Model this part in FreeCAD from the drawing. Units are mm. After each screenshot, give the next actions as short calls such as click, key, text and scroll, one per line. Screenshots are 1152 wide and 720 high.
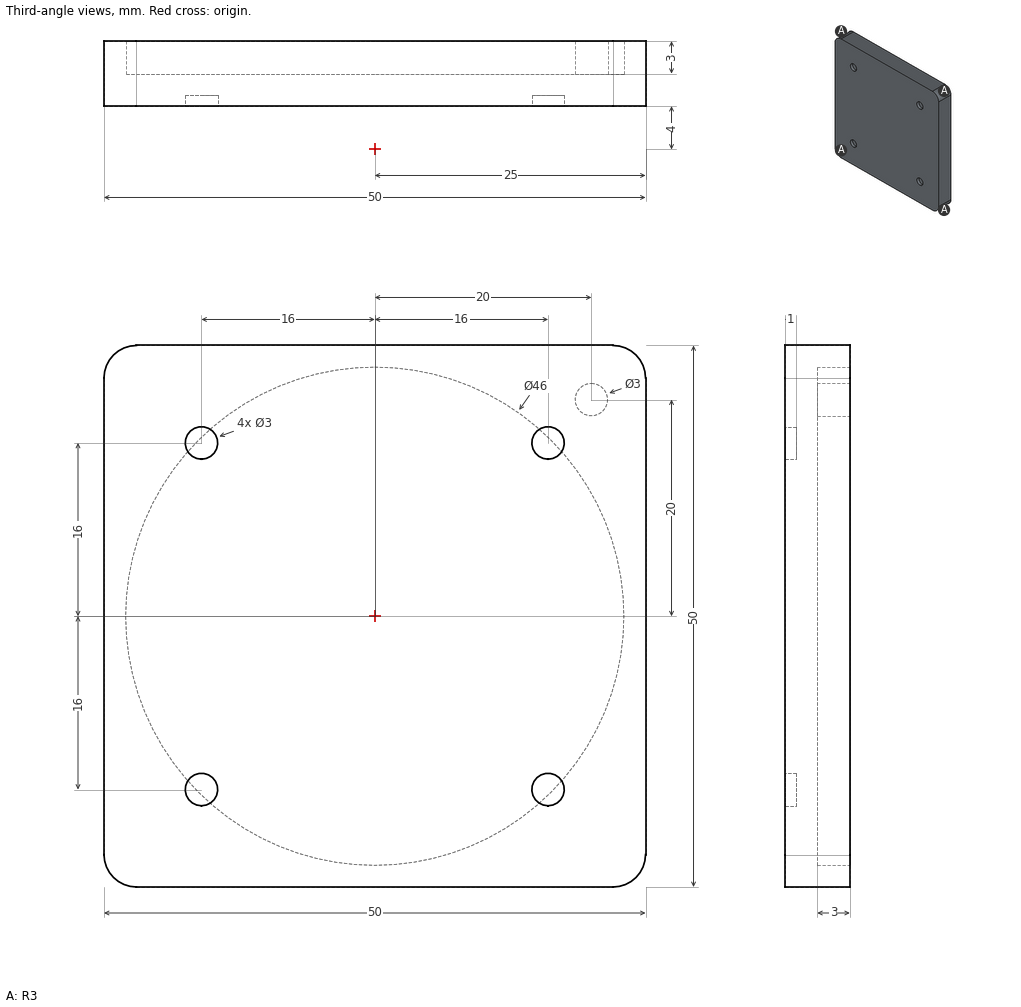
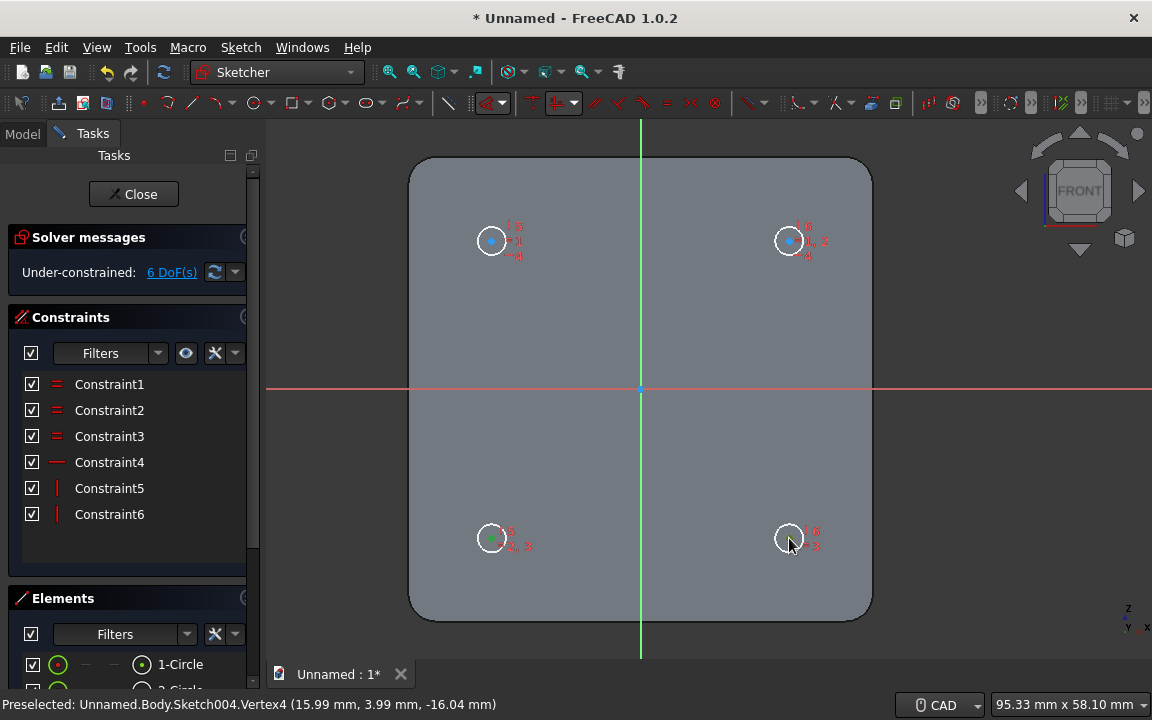
click(576, 104)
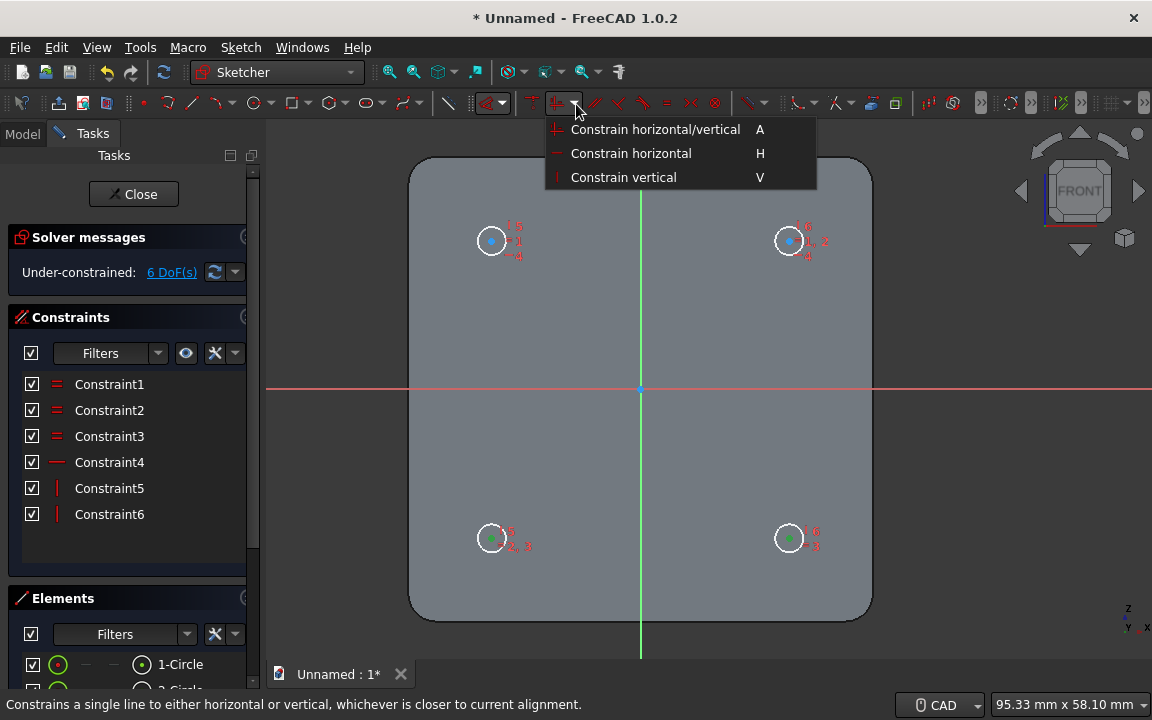
click(681, 153)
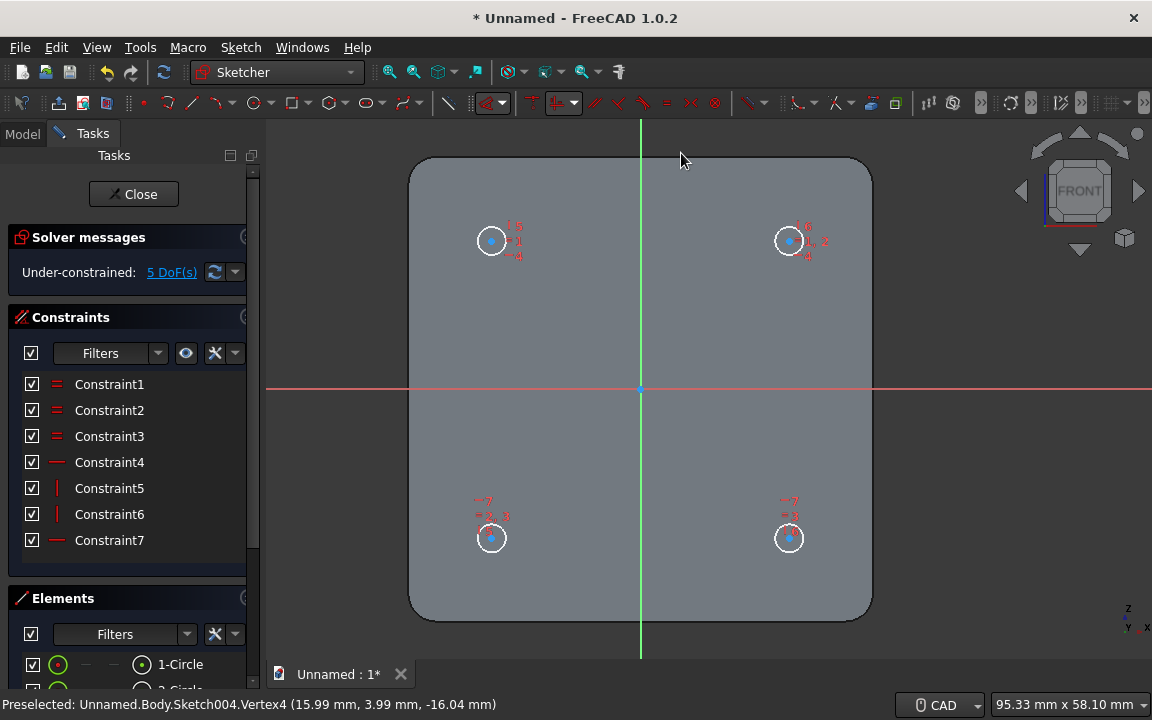
scroll(502, 231, up, 2)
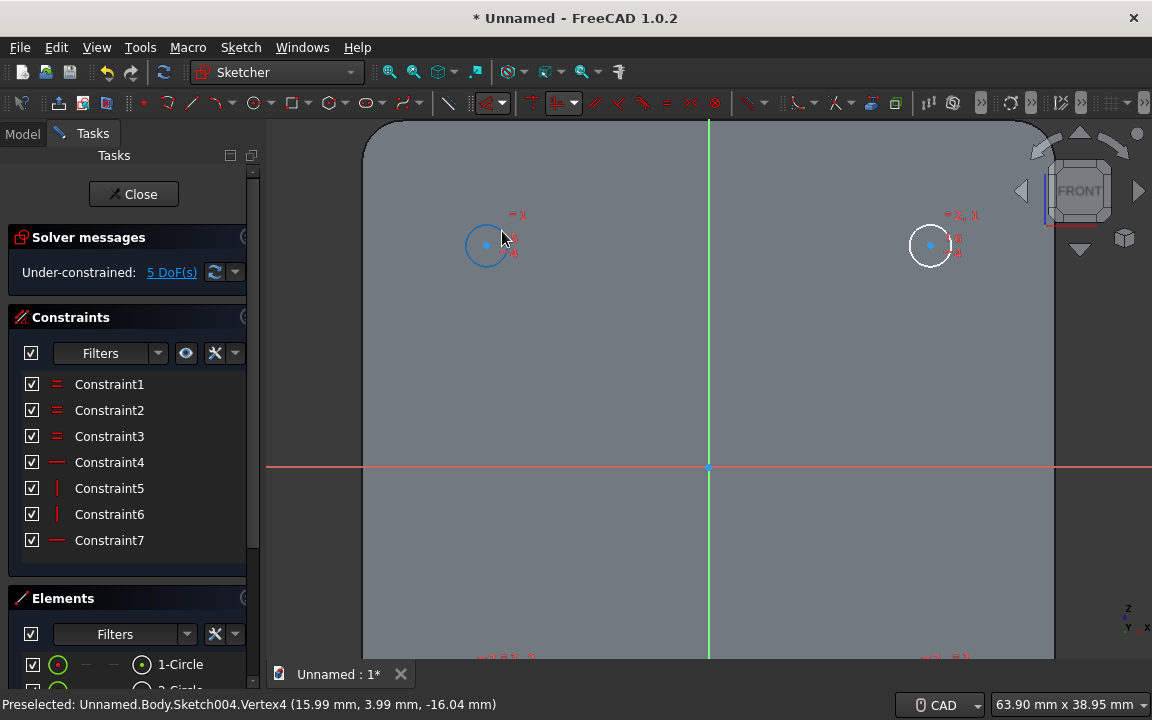
click(472, 231)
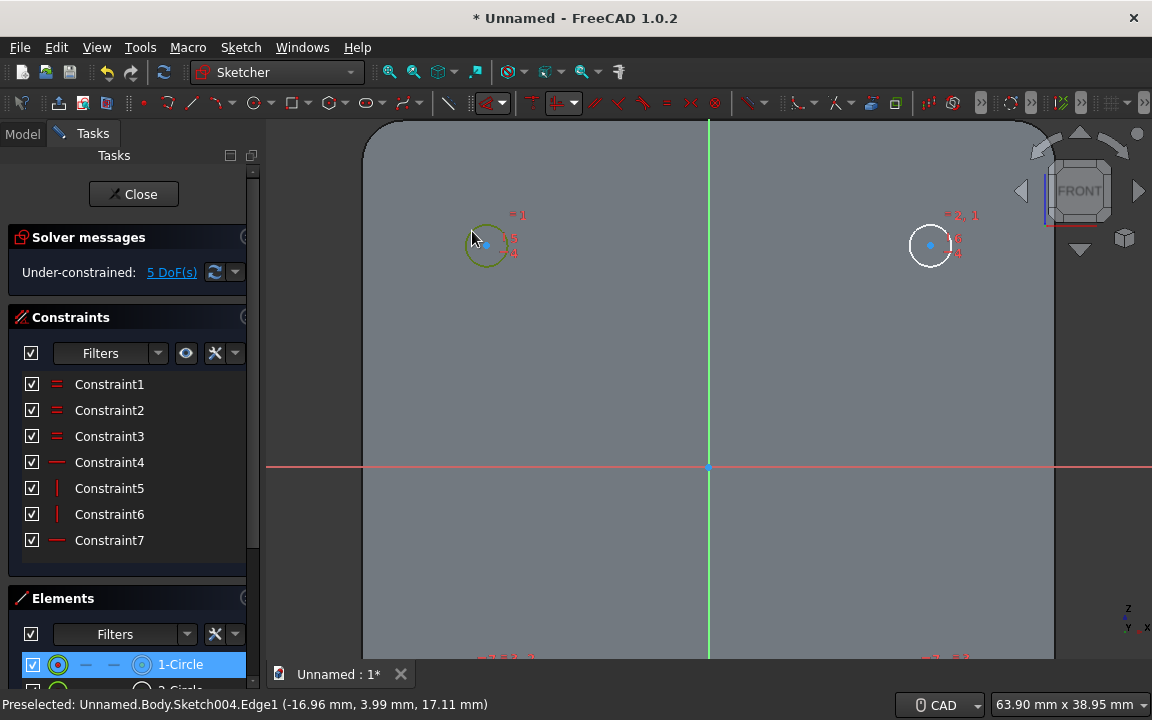
key(k)
key(o)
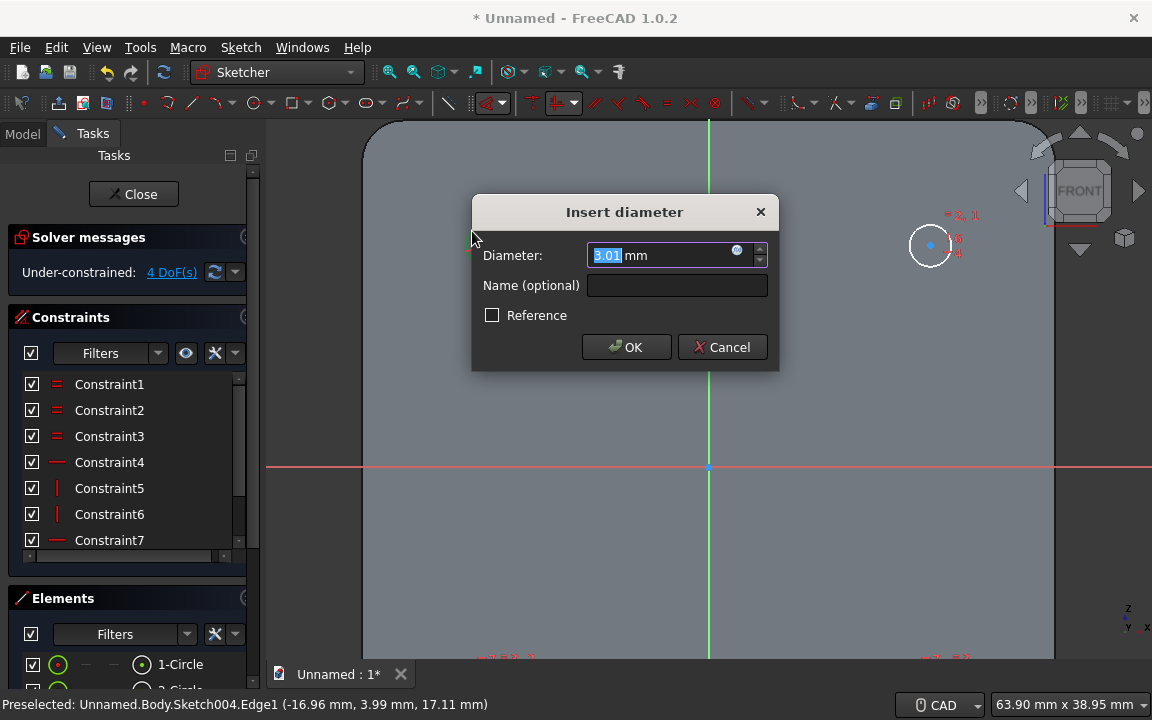
text(3)
key(Return)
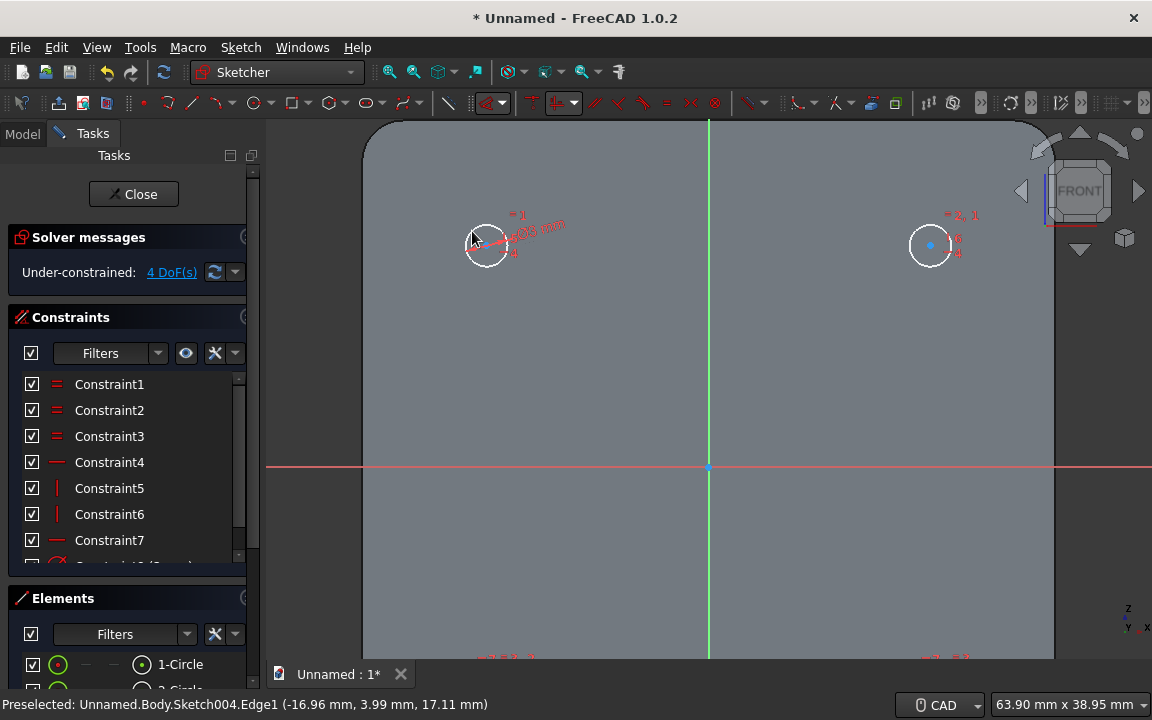
click(487, 246)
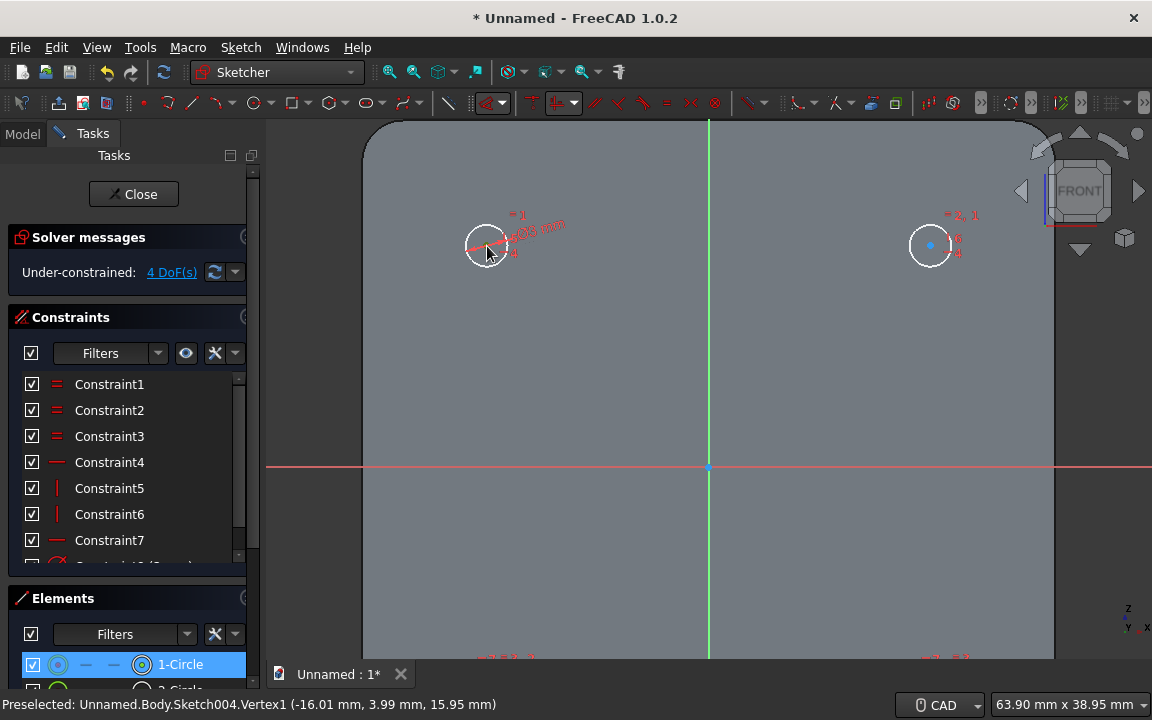
click(504, 104)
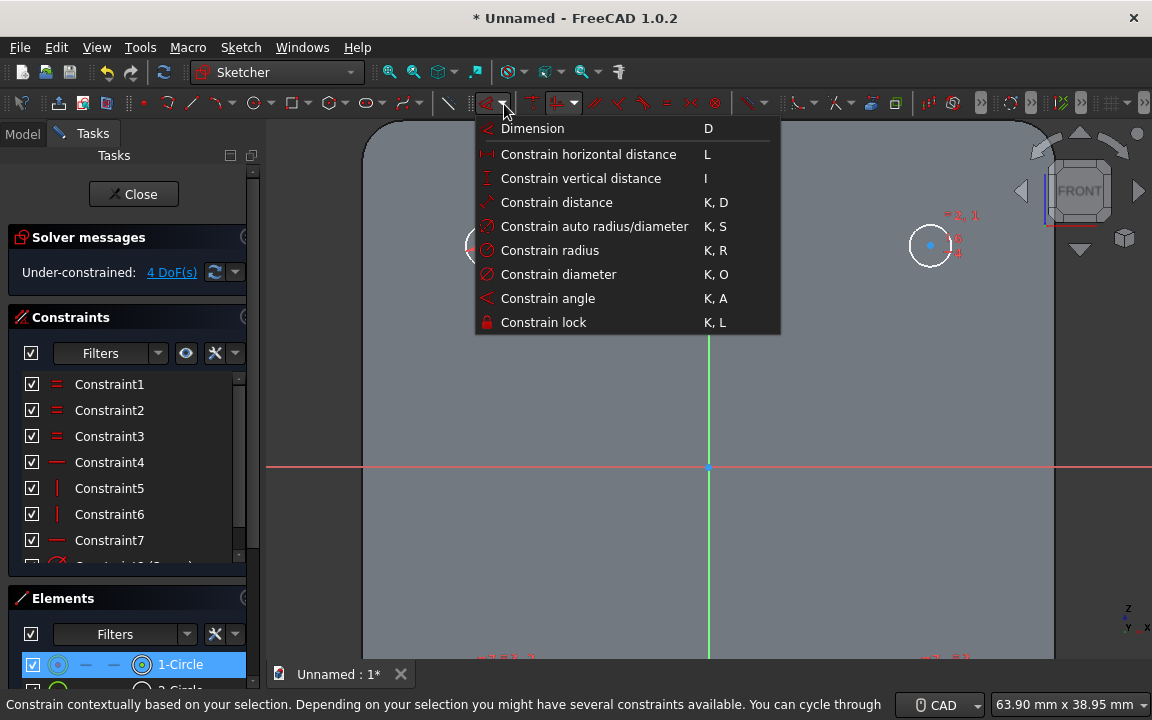
click(628, 154)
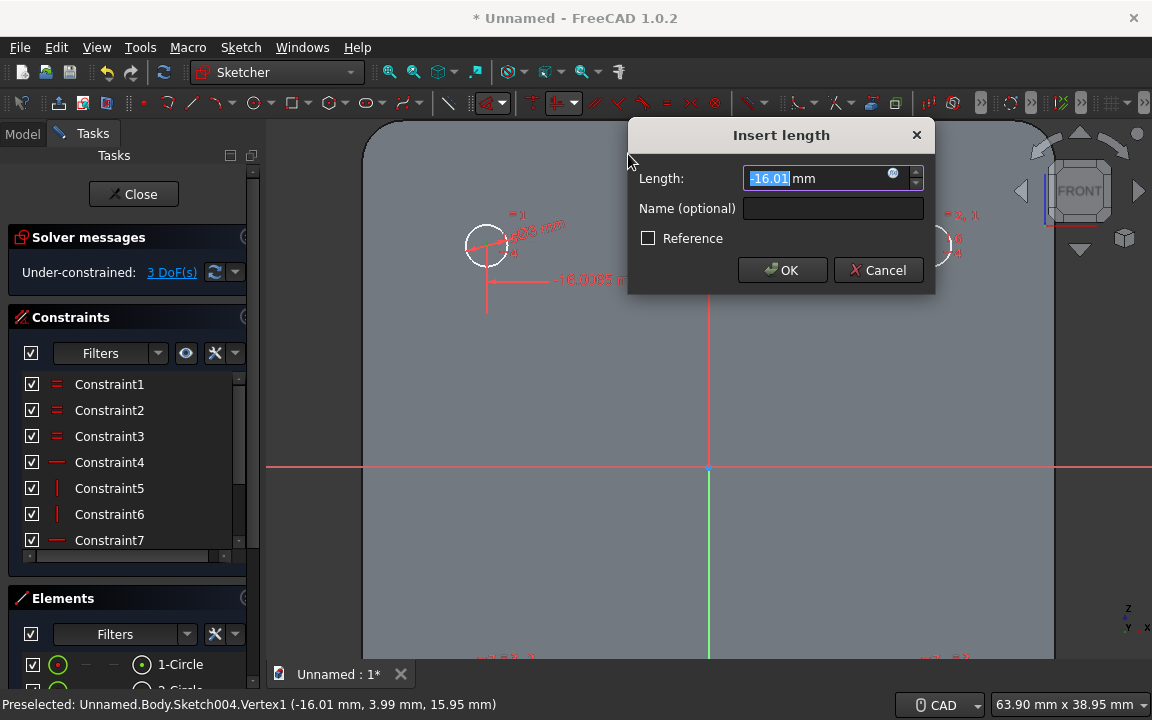
text(-16)
key(Return)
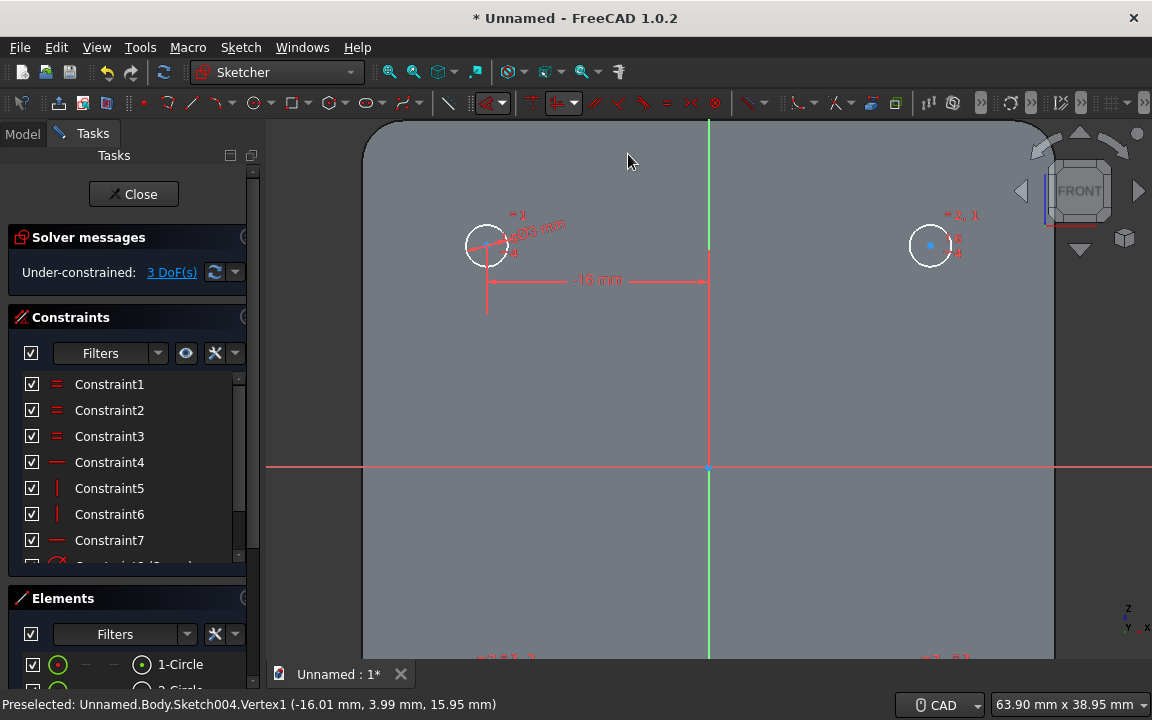
click(487, 246)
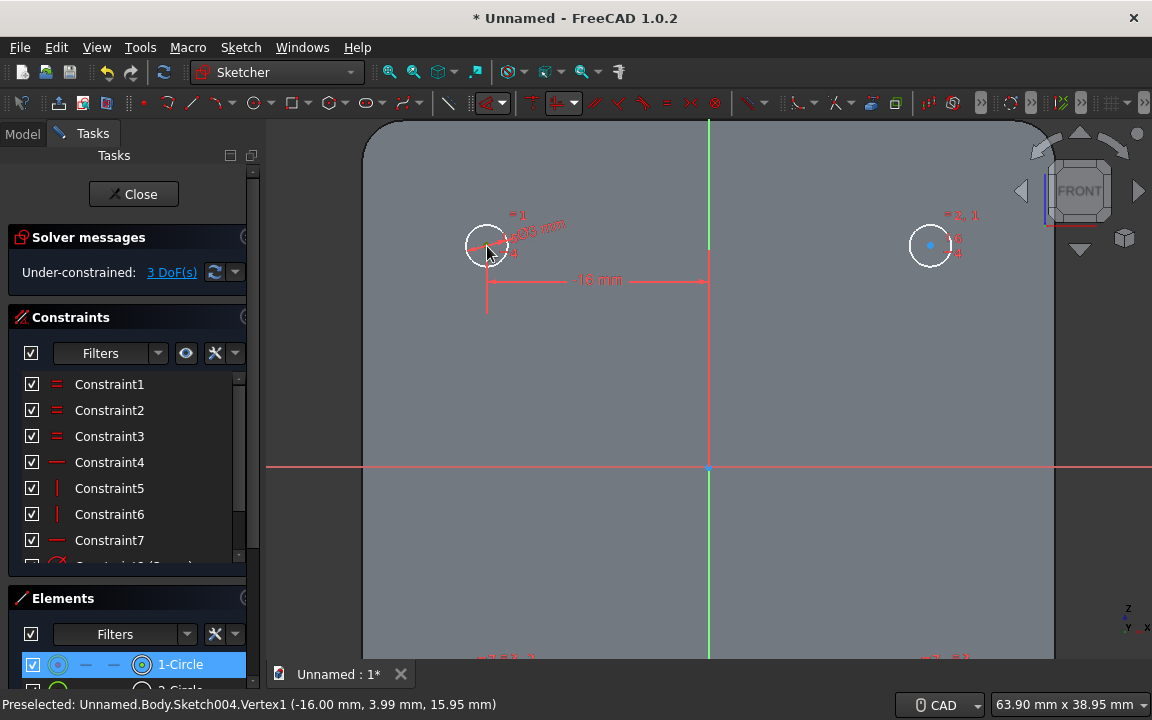
click(504, 104)